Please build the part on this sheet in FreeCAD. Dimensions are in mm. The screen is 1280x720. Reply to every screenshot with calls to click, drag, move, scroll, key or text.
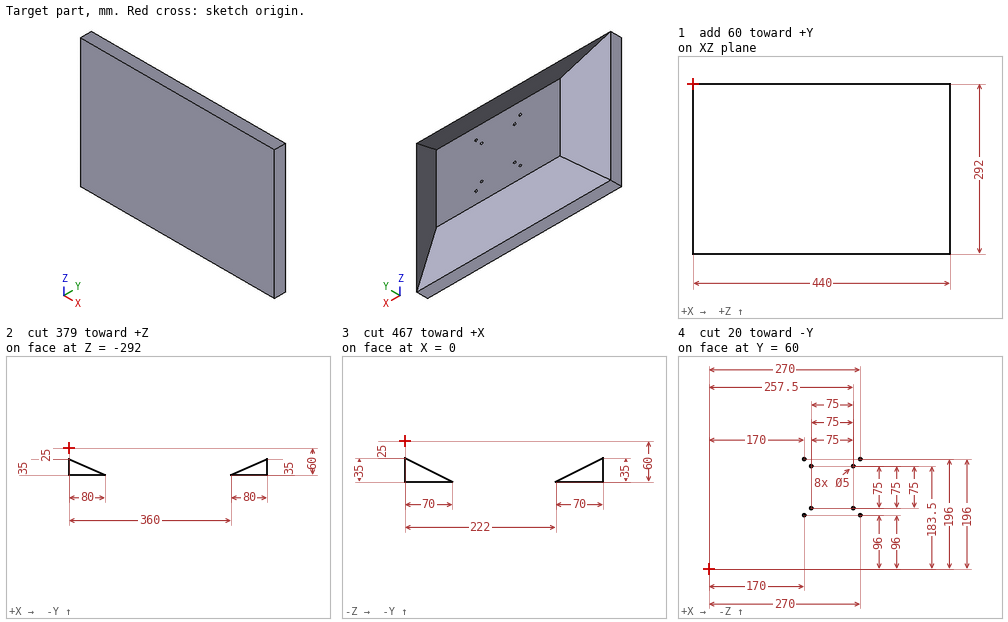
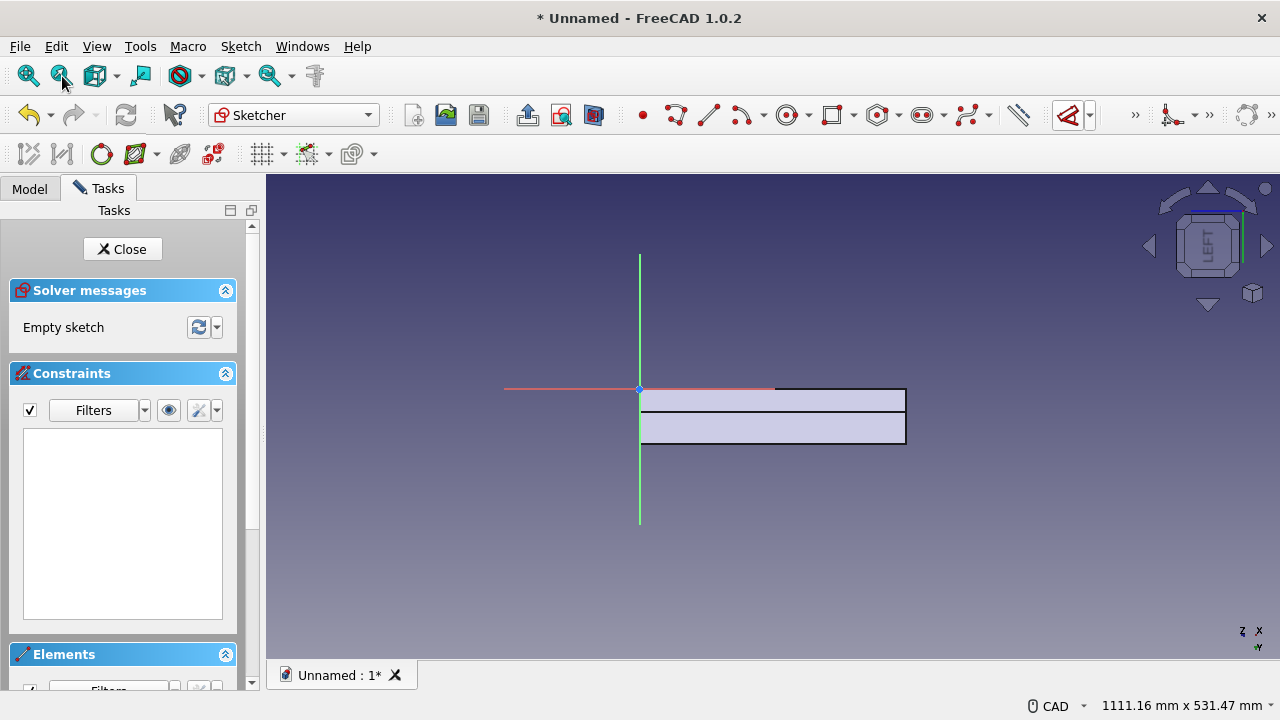
scroll(829, 416, up, 4)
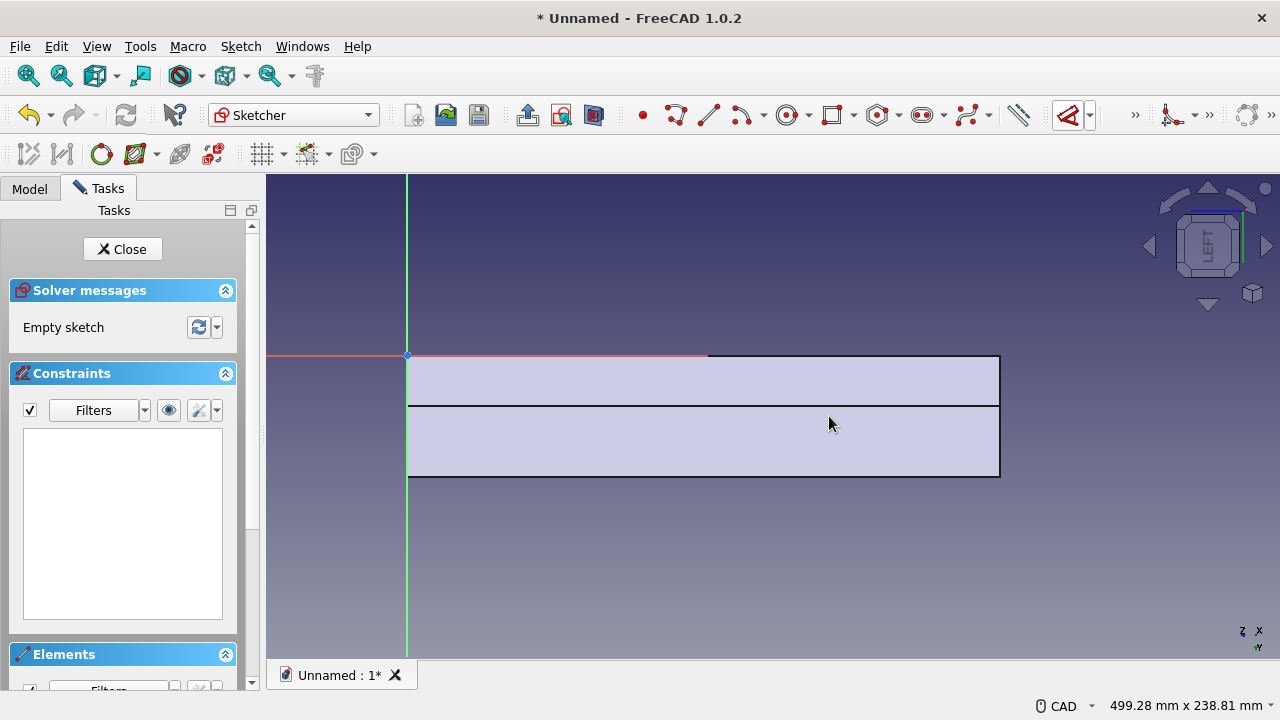
click(676, 116)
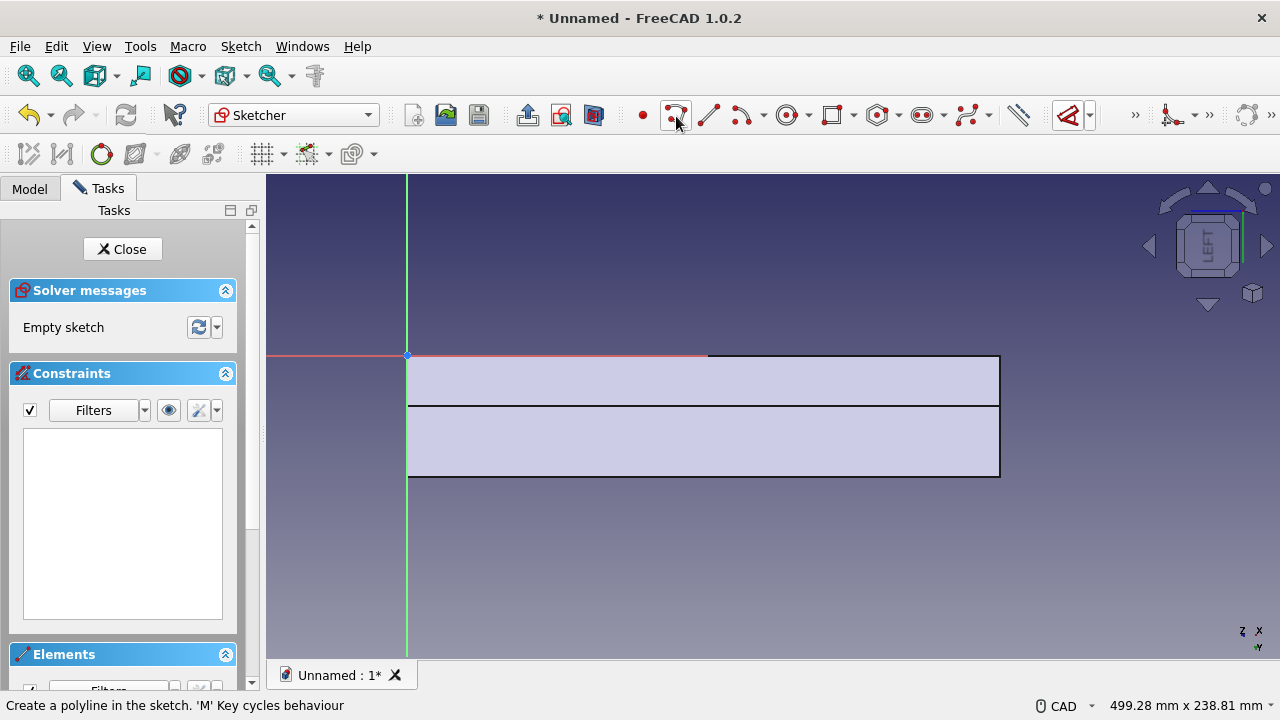
click(858, 477)
click(1000, 477)
click(1000, 406)
click(858, 478)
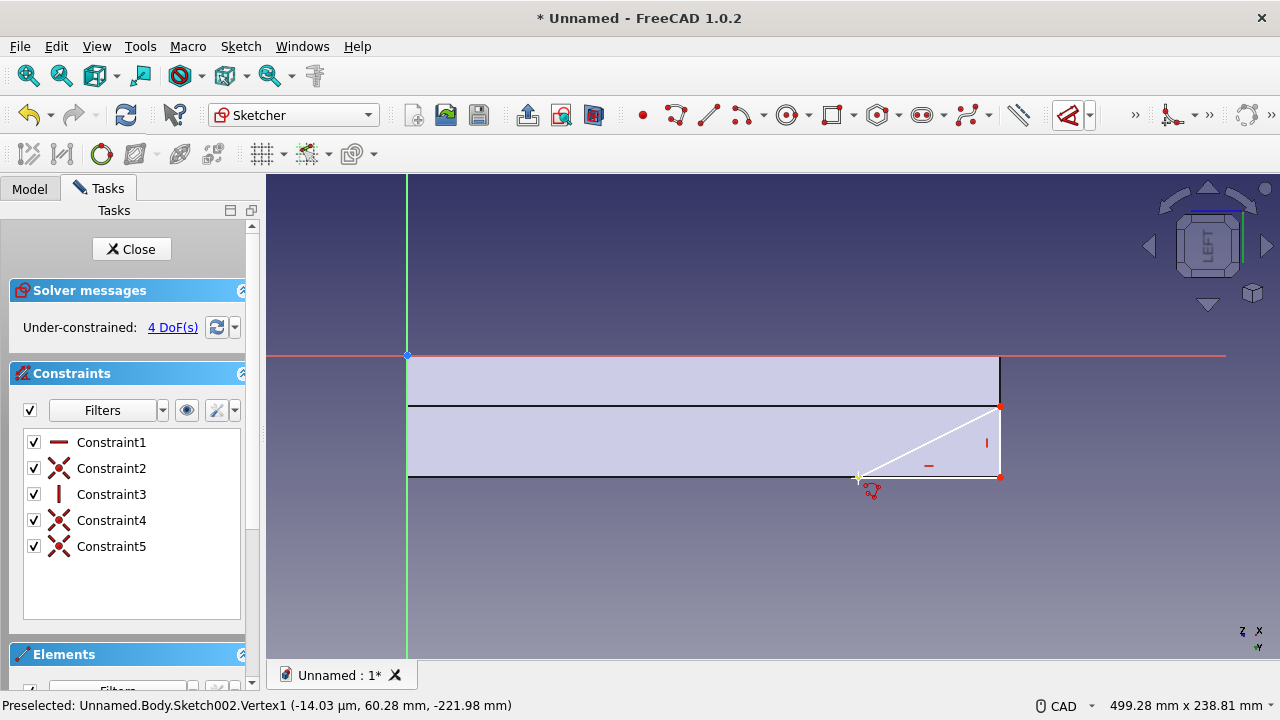
click(407, 406)
click(416, 477)
click(549, 477)
click(407, 407)
key(Escape)
key(Escape)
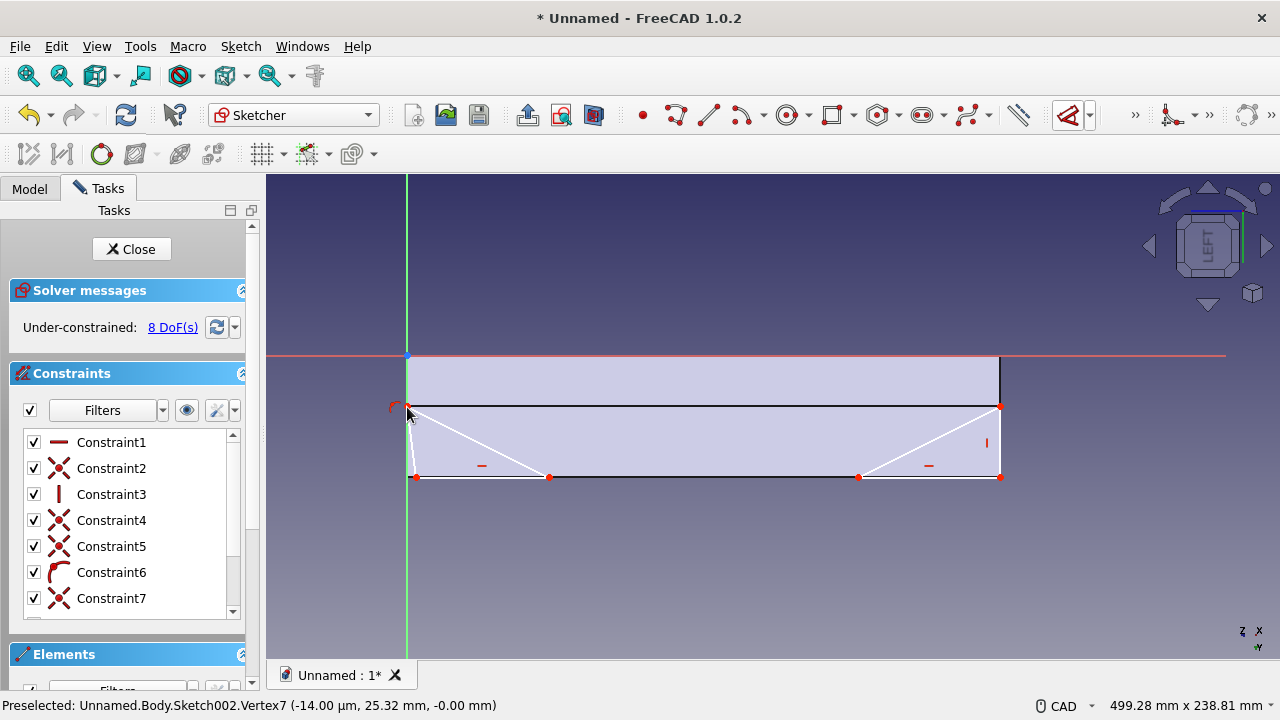
click(410, 428)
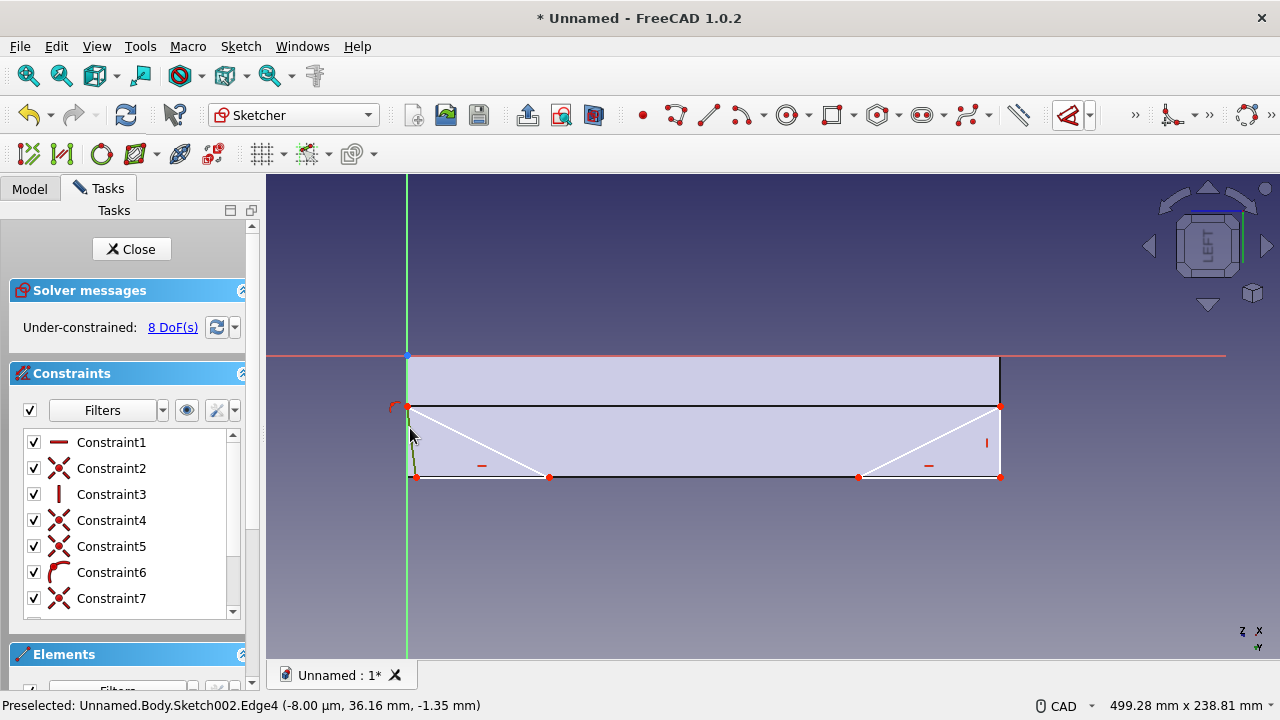
key(v)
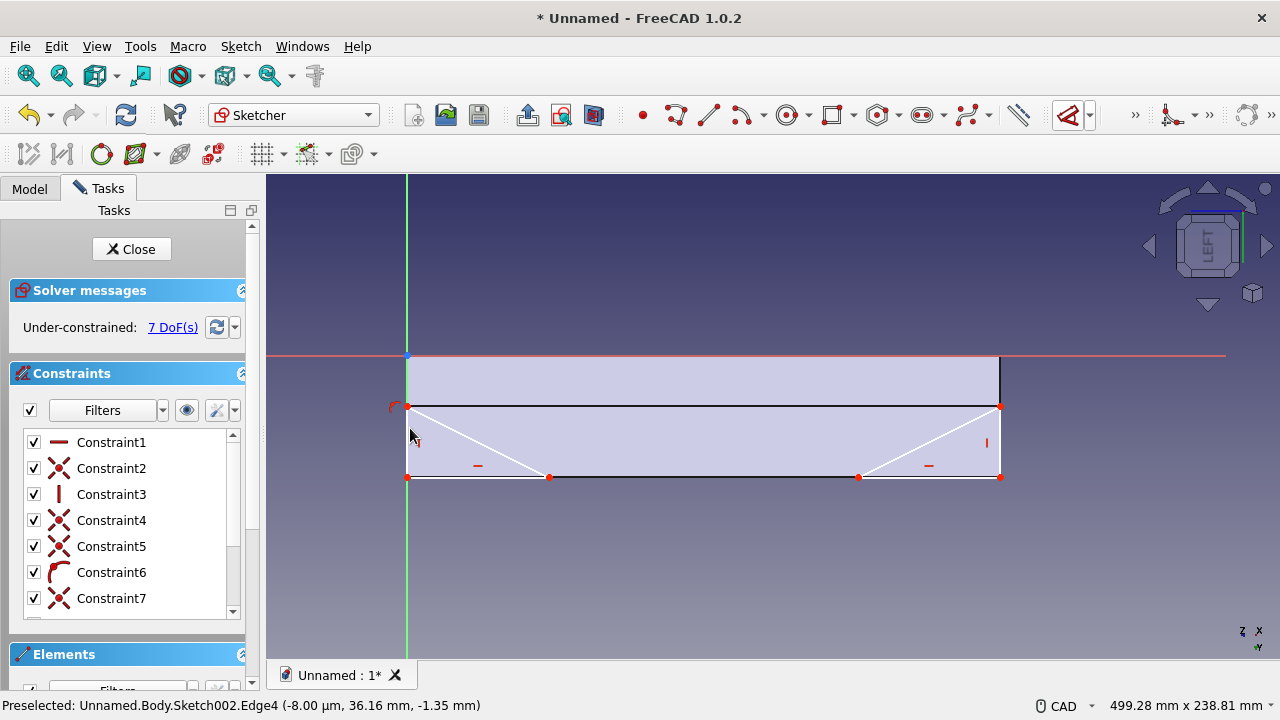
click(901, 478)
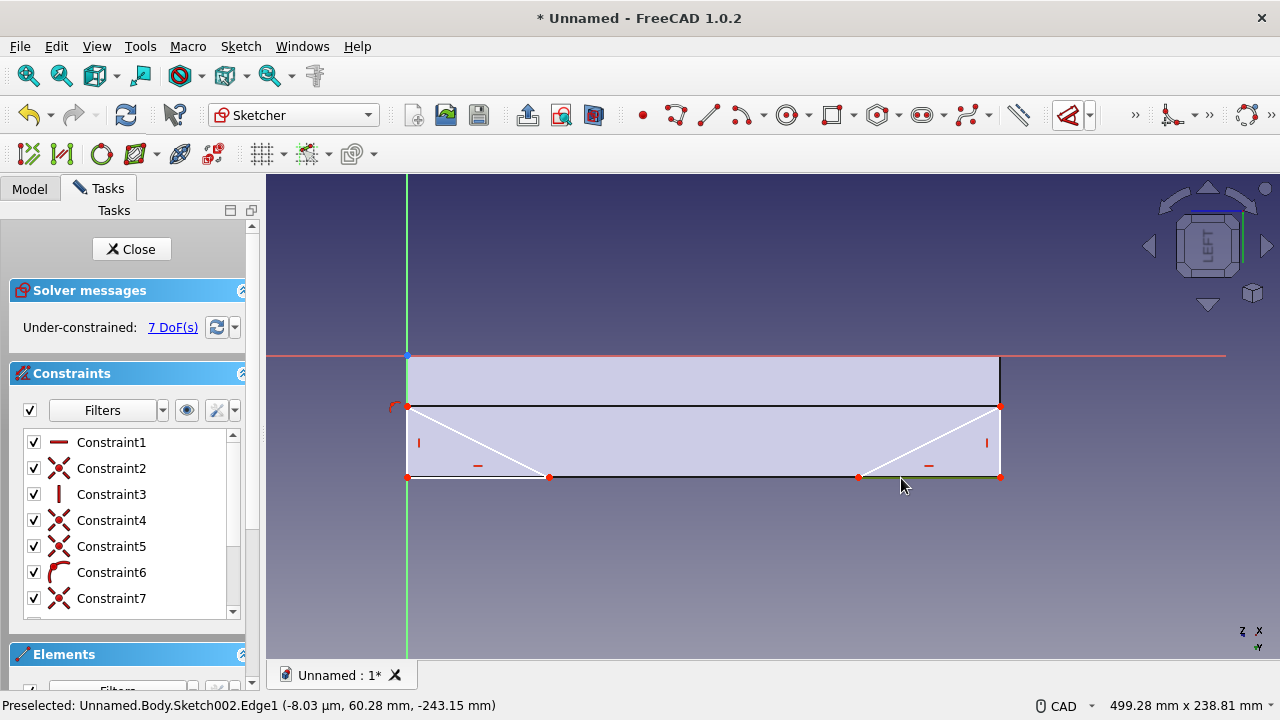
key(l)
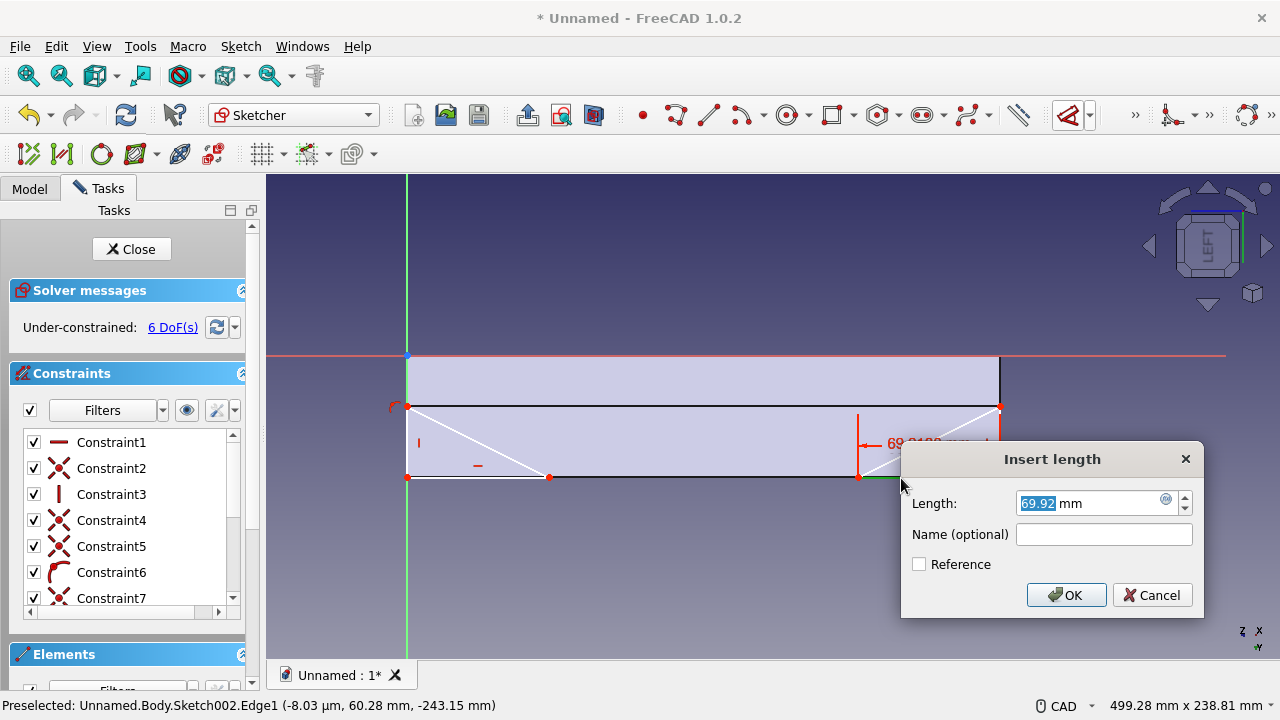
text(70)
key(Return)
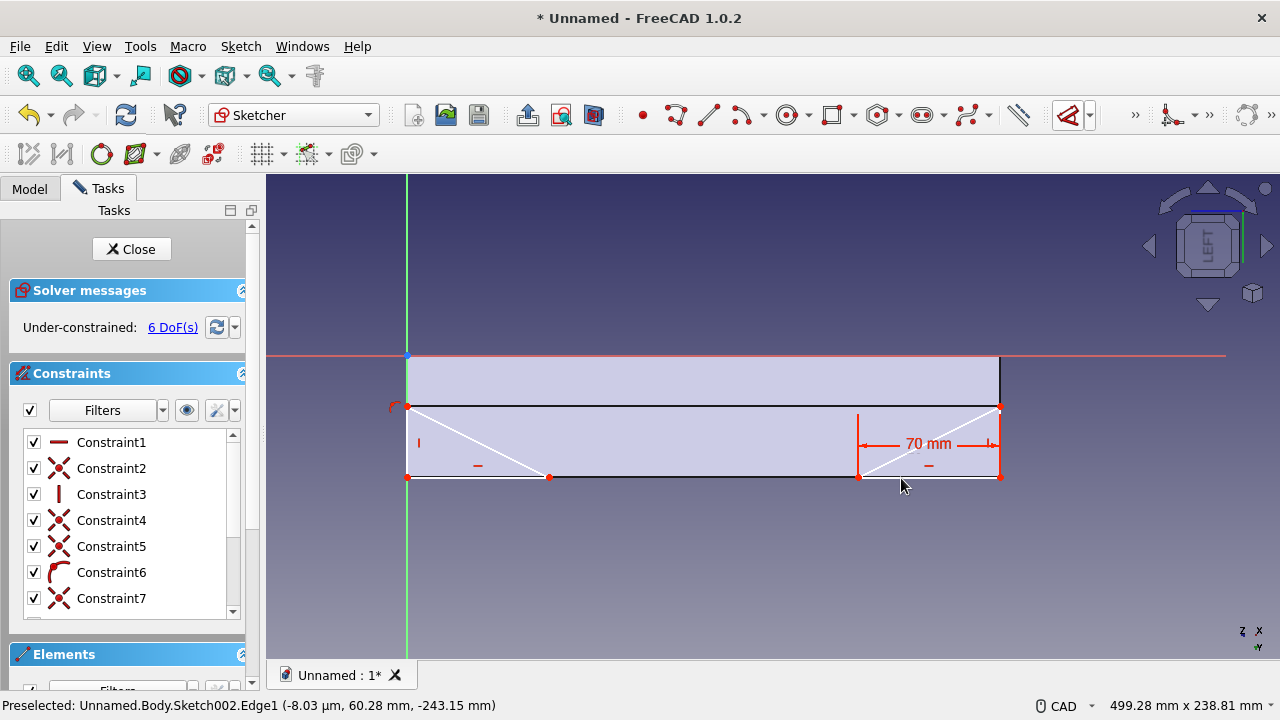
click(1000, 457)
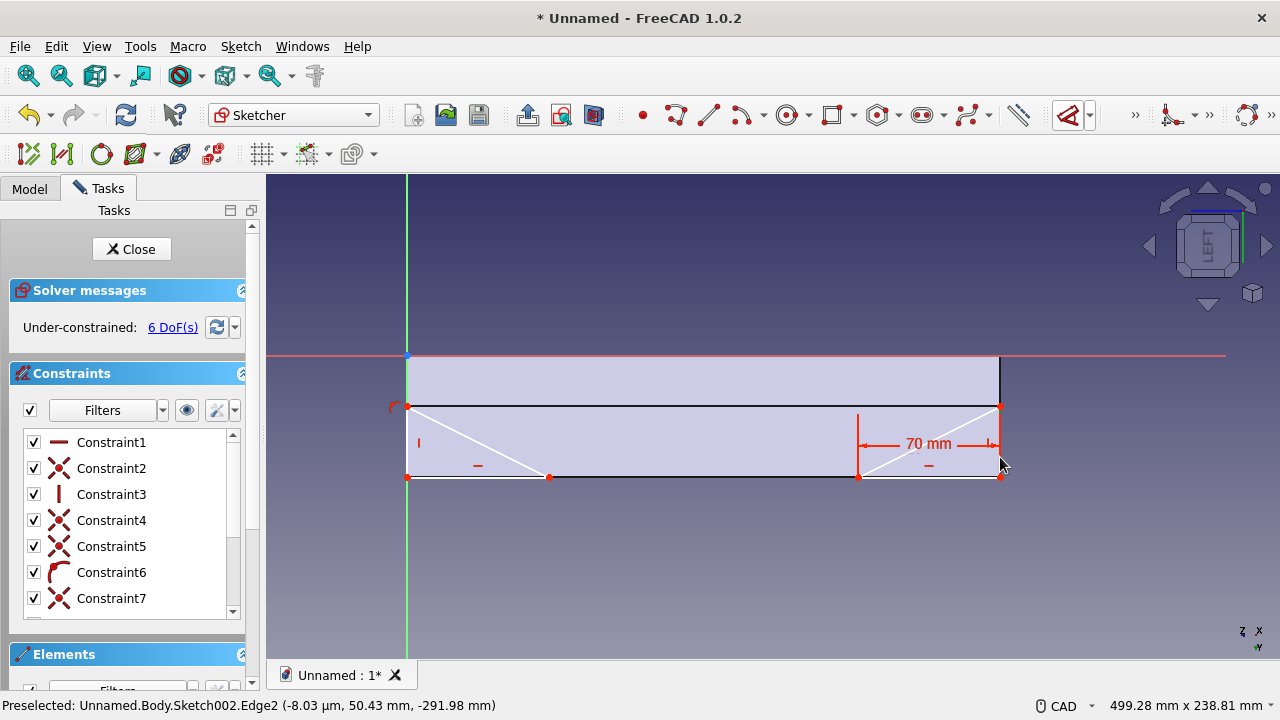
key(i)